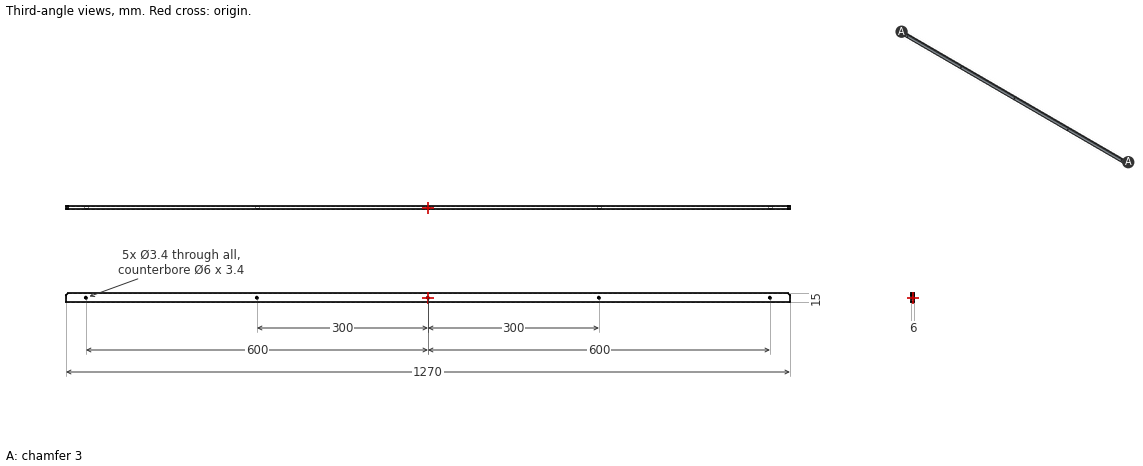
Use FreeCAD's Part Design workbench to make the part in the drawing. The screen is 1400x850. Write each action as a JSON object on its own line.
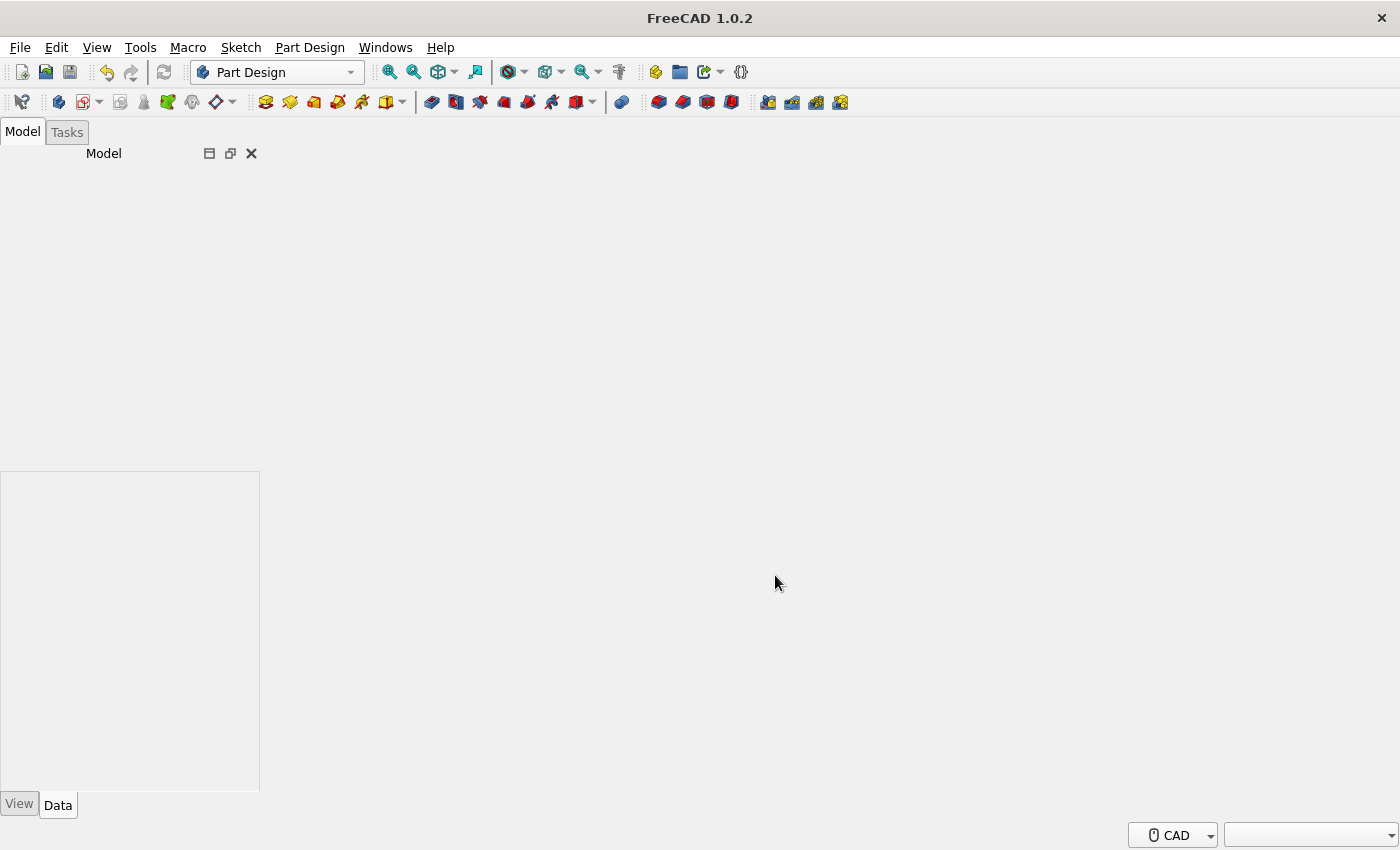
{"action": "left_click", "coordinate": [22, 72]}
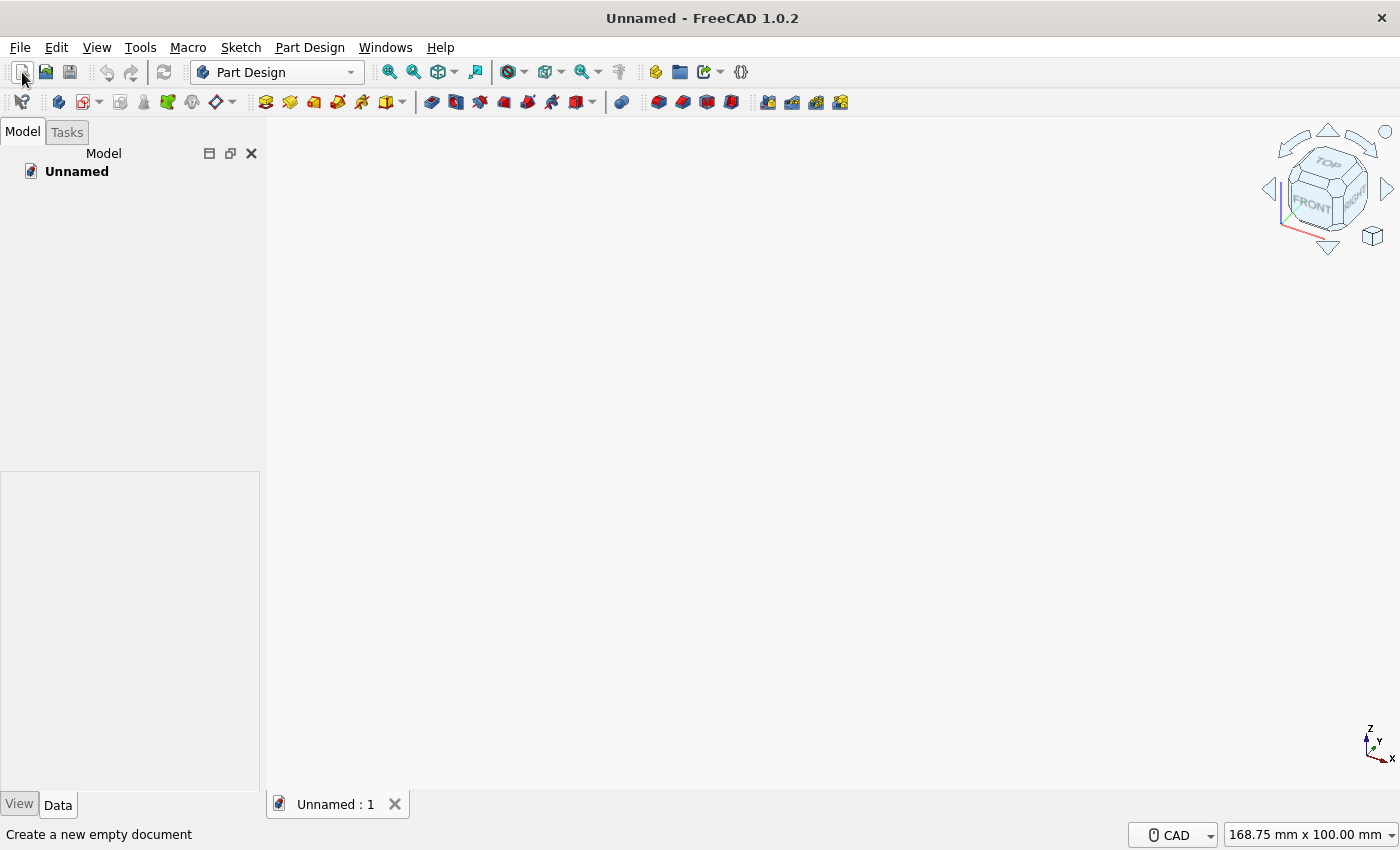
{"action": "left_click", "coordinate": [84, 102]}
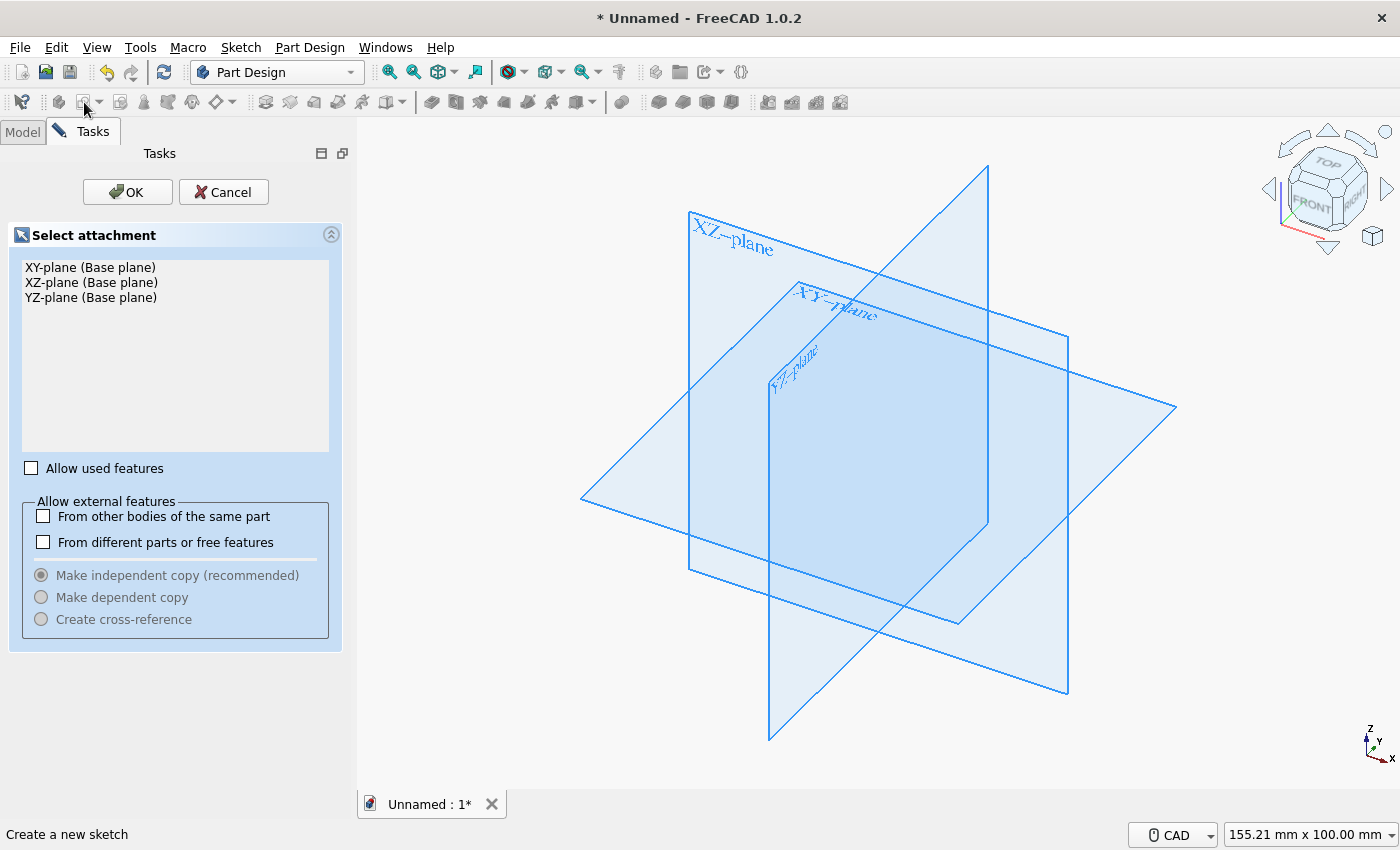
{"action": "left_click", "coordinate": [82, 282]}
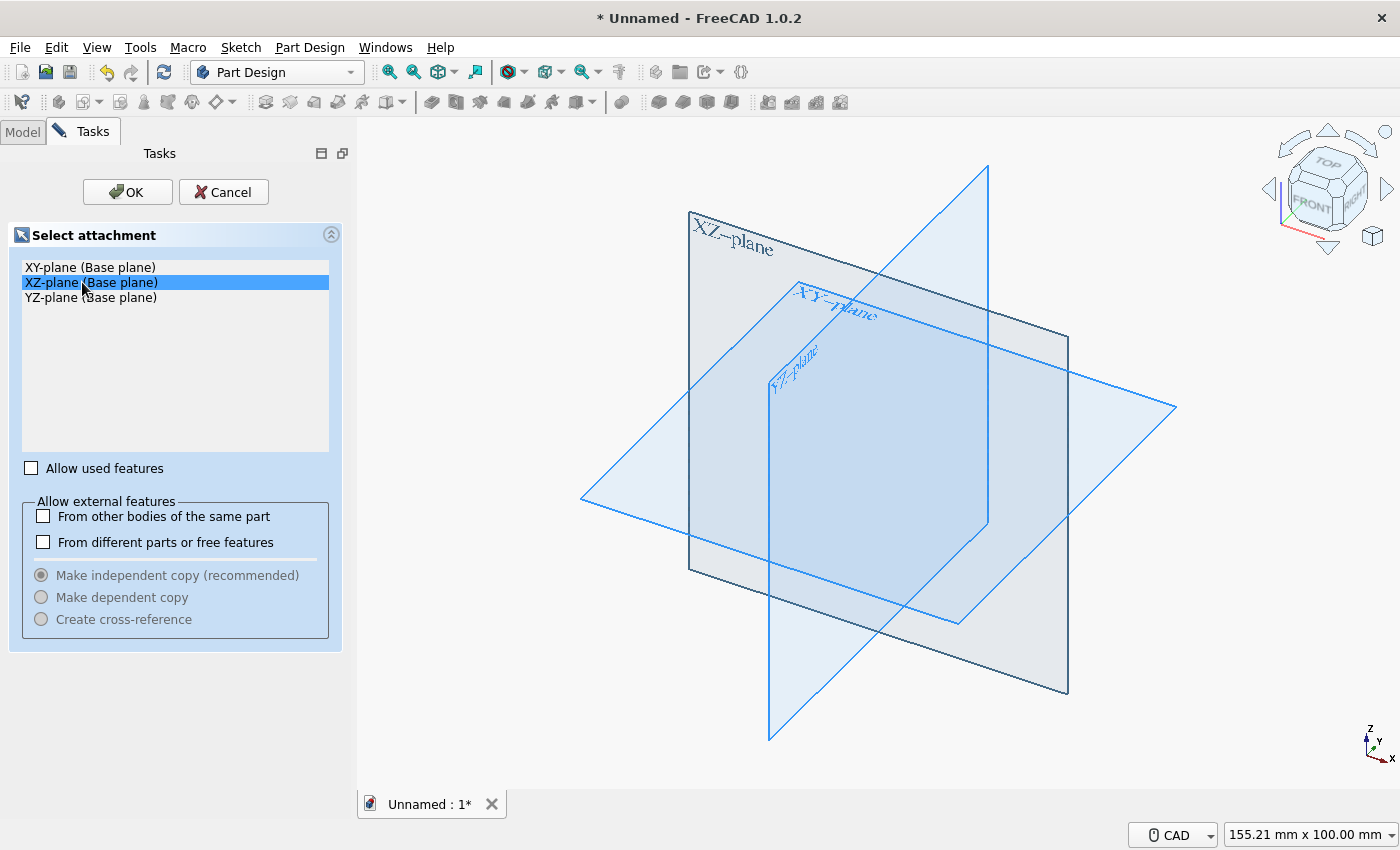
{"action": "left_click", "coordinate": [128, 192]}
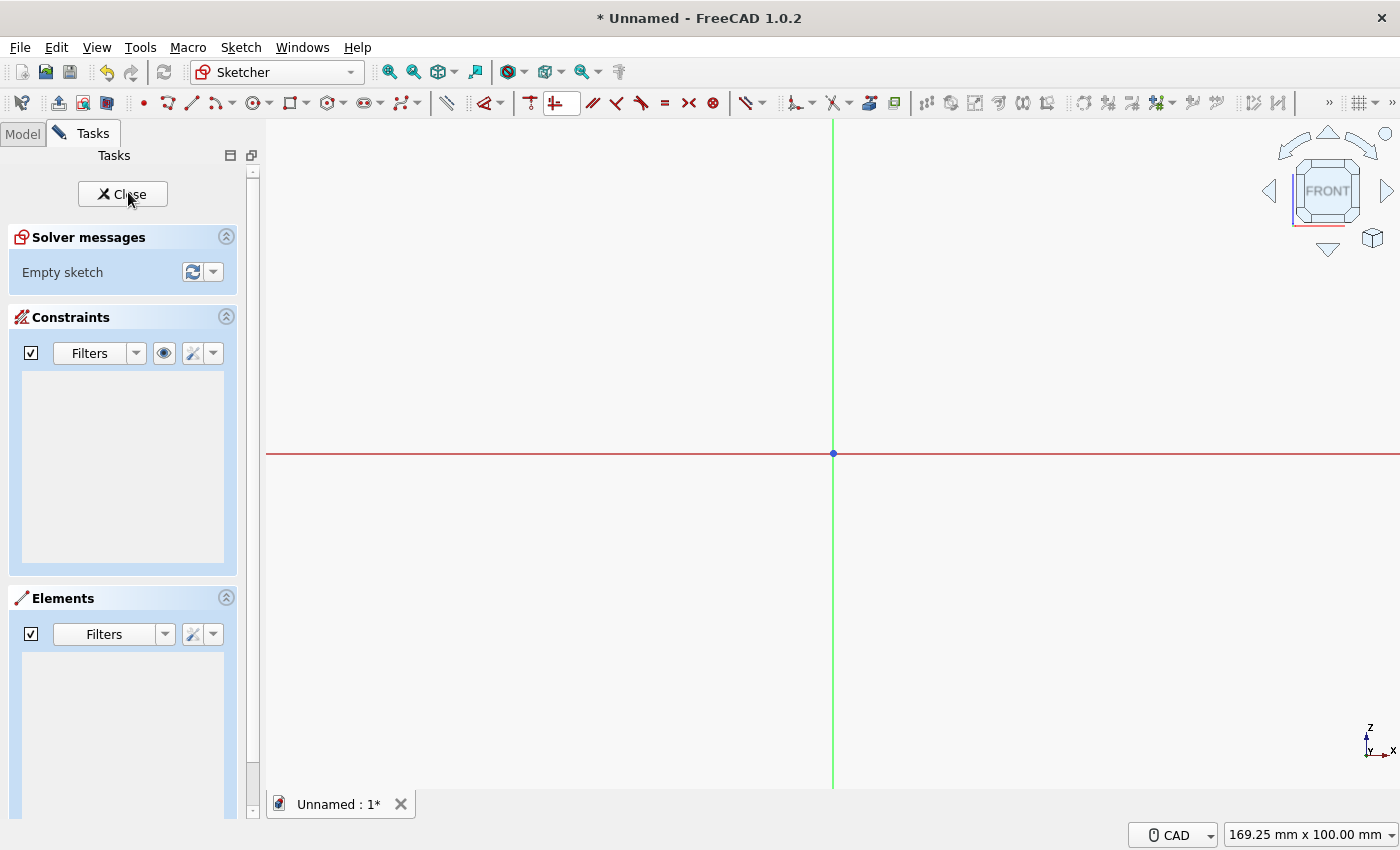
{"action": "scroll", "coordinate": [759, 454], "scroll_direction": "down", "scroll_amount": 13}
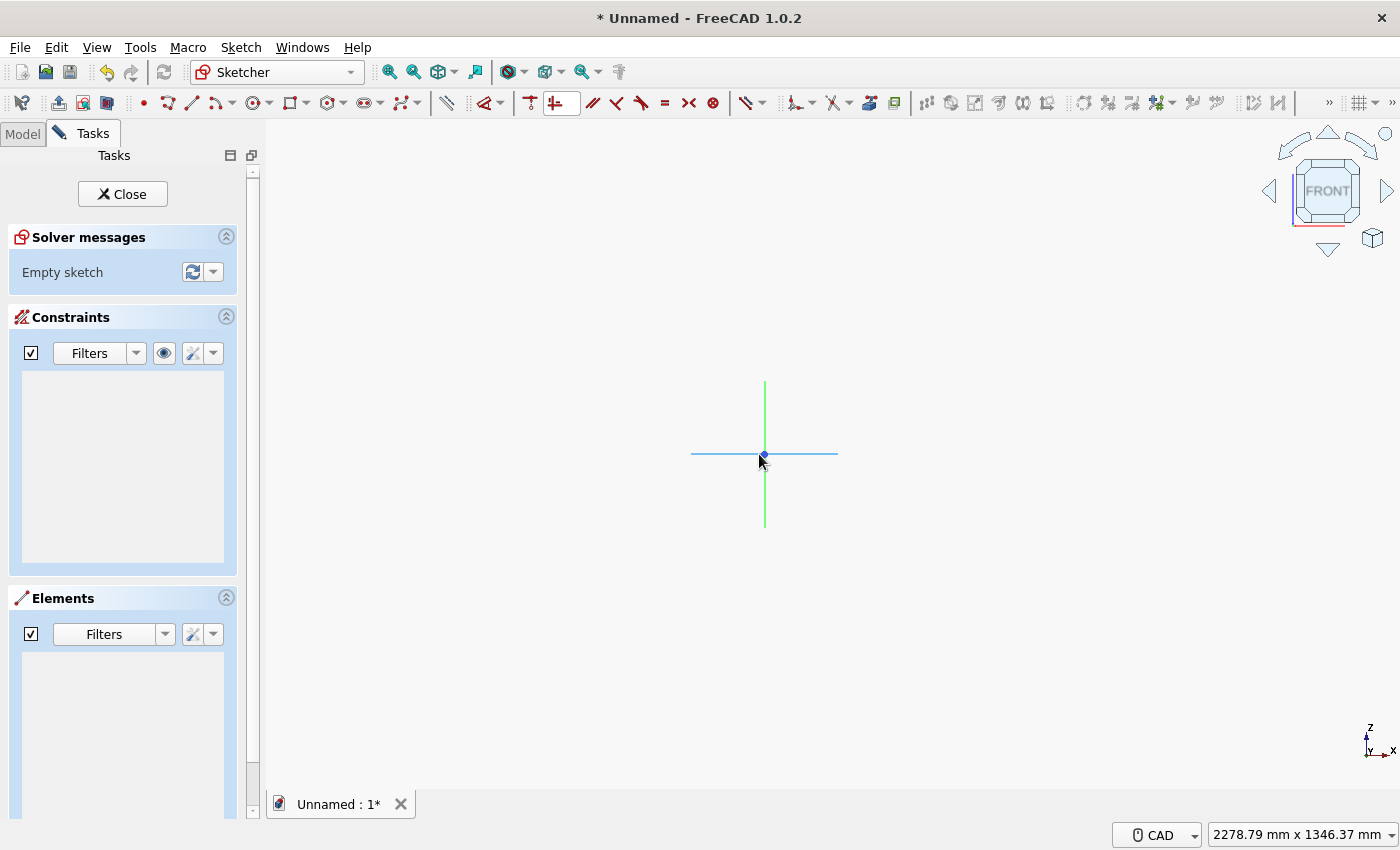
{"action": "key", "text": "g v"}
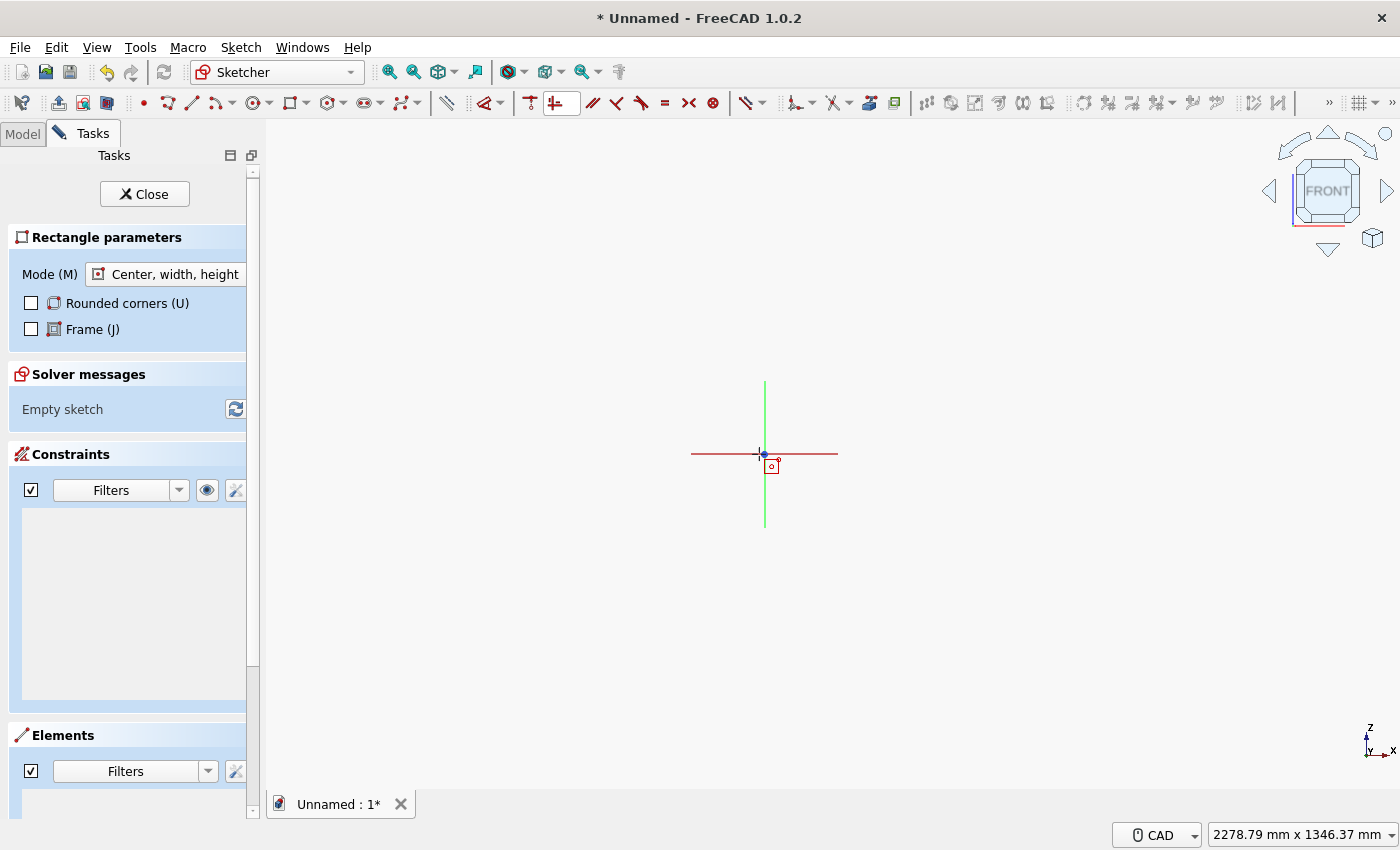
{"action": "scroll", "coordinate": [765, 454], "scroll_direction": "up", "scroll_amount": 8}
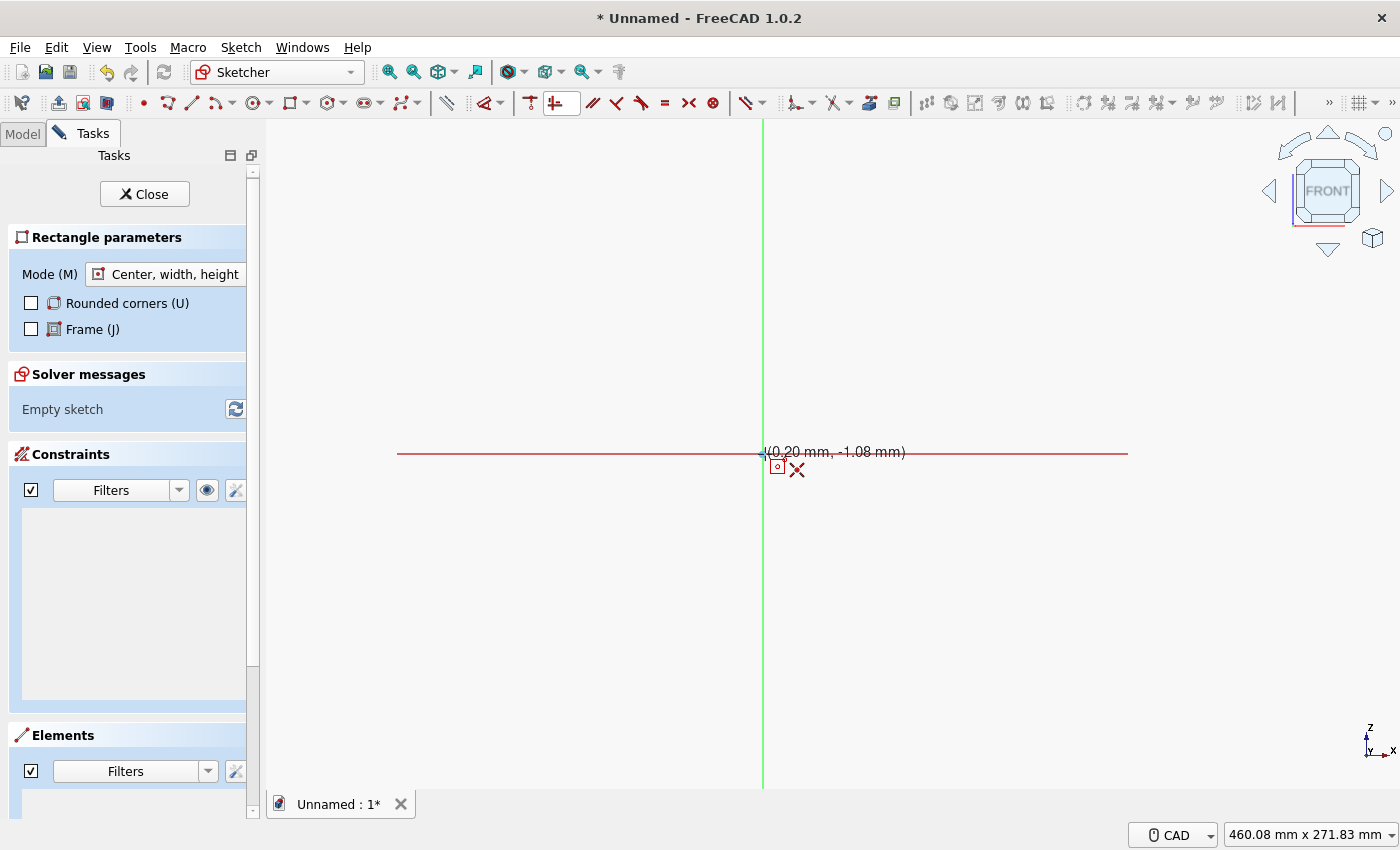
{"action": "scroll", "coordinate": [765, 454], "scroll_direction": "down", "scroll_amount": 8}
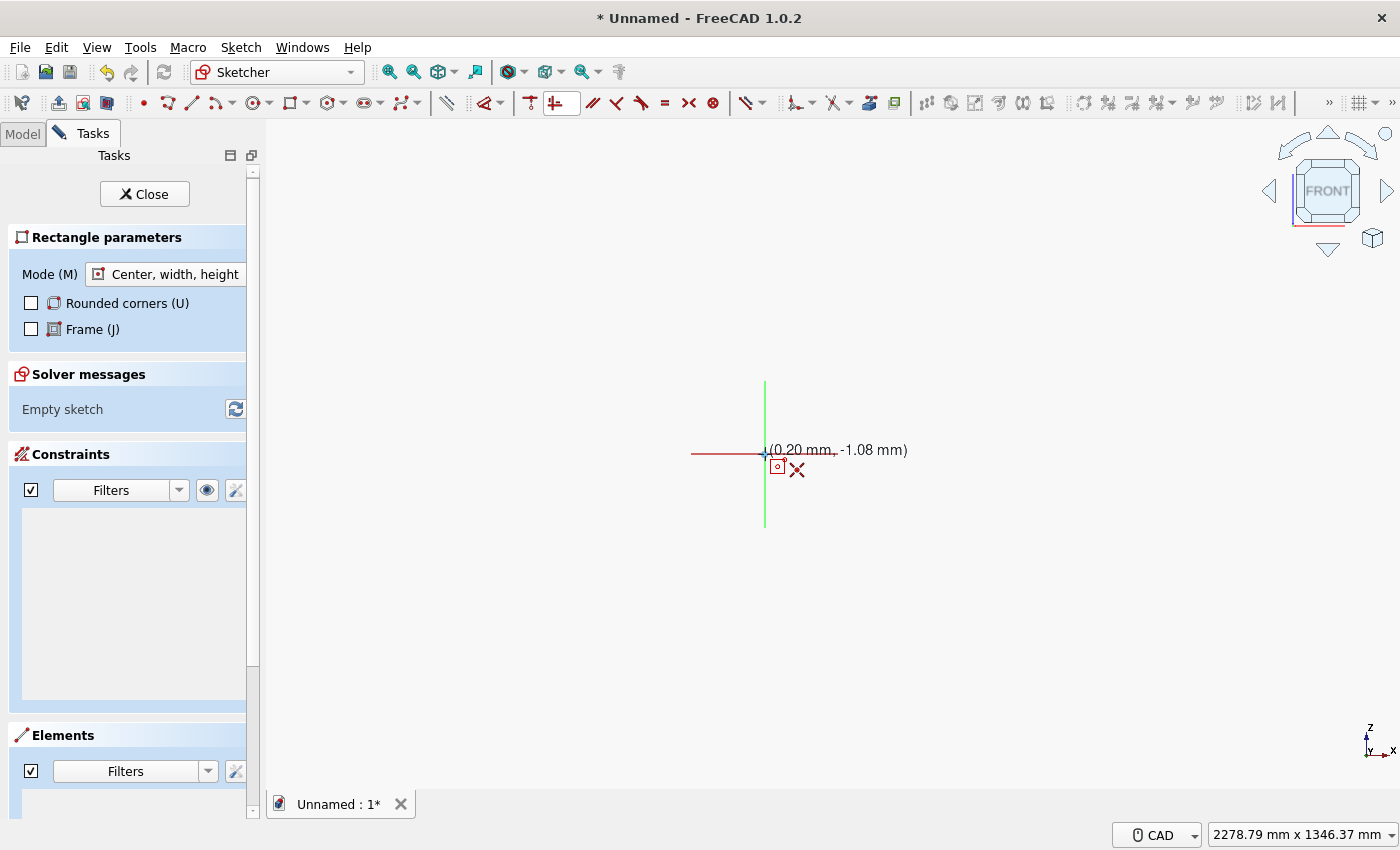
{"action": "left_click", "coordinate": [765, 454]}